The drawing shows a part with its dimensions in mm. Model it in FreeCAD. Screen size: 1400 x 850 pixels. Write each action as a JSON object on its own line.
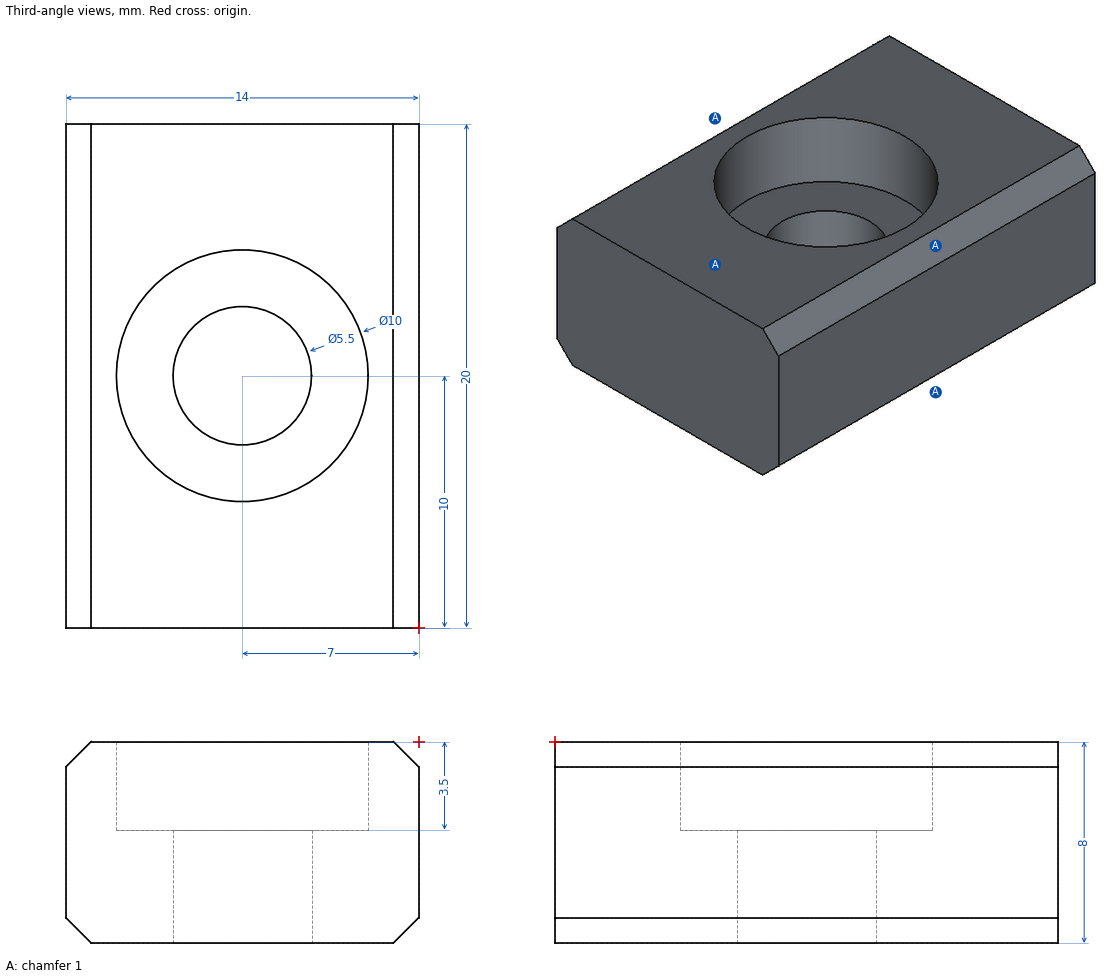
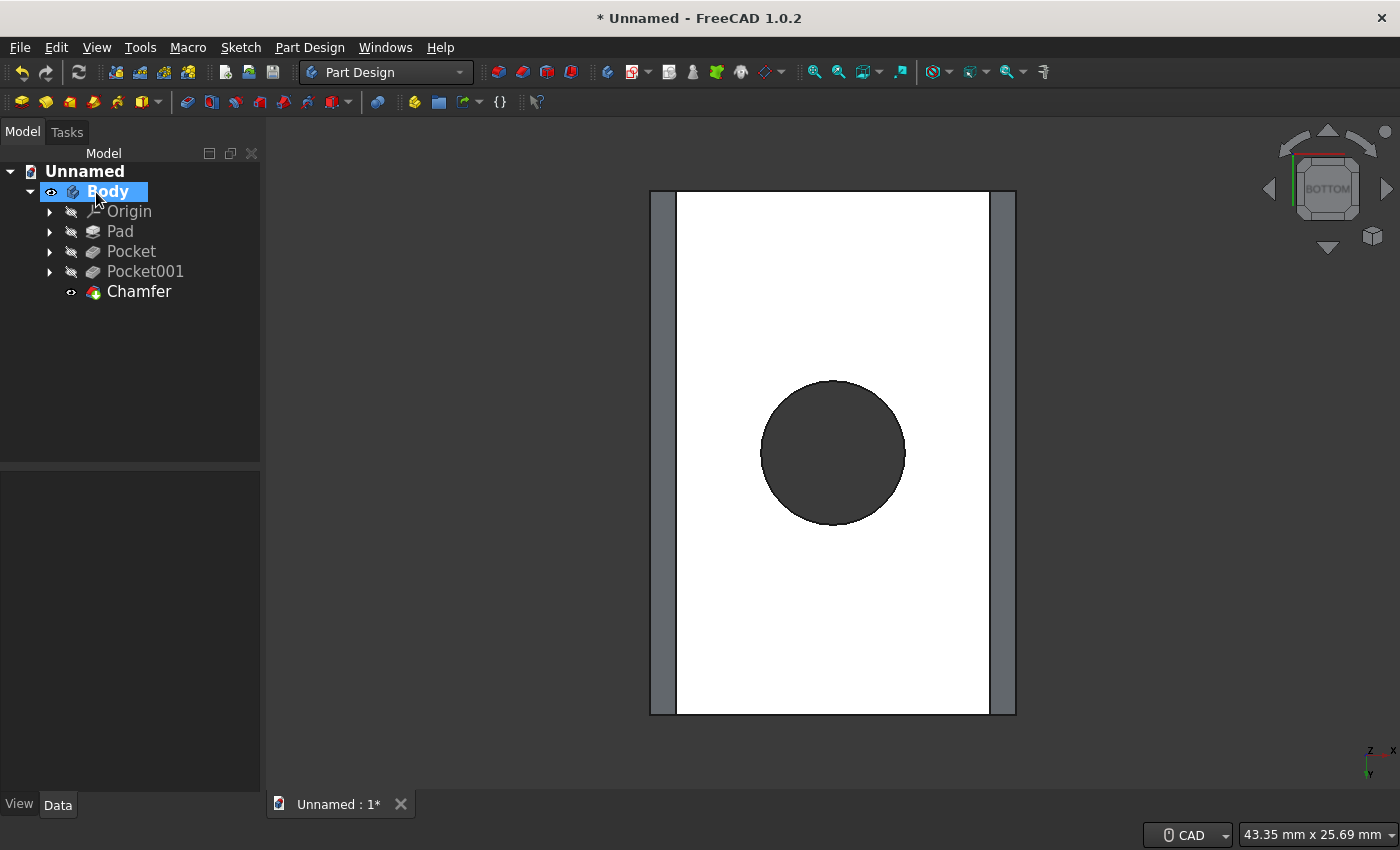
{"action": "key", "text": "0"}